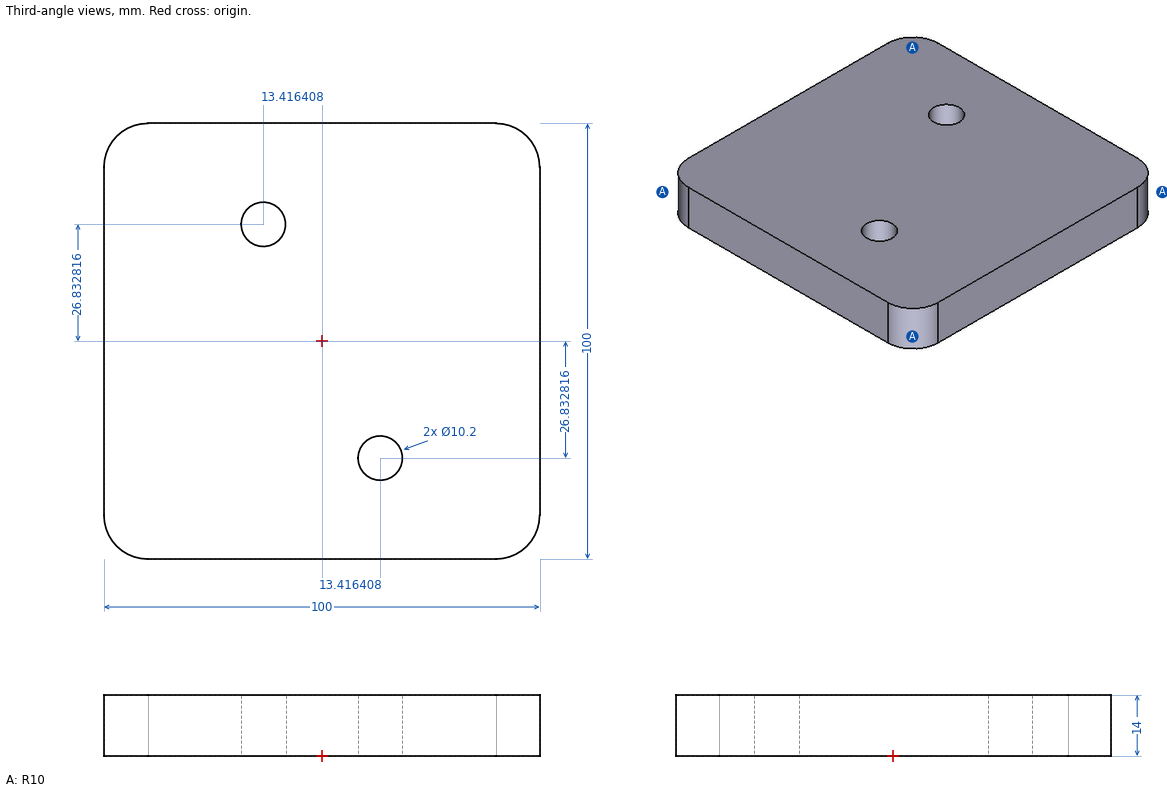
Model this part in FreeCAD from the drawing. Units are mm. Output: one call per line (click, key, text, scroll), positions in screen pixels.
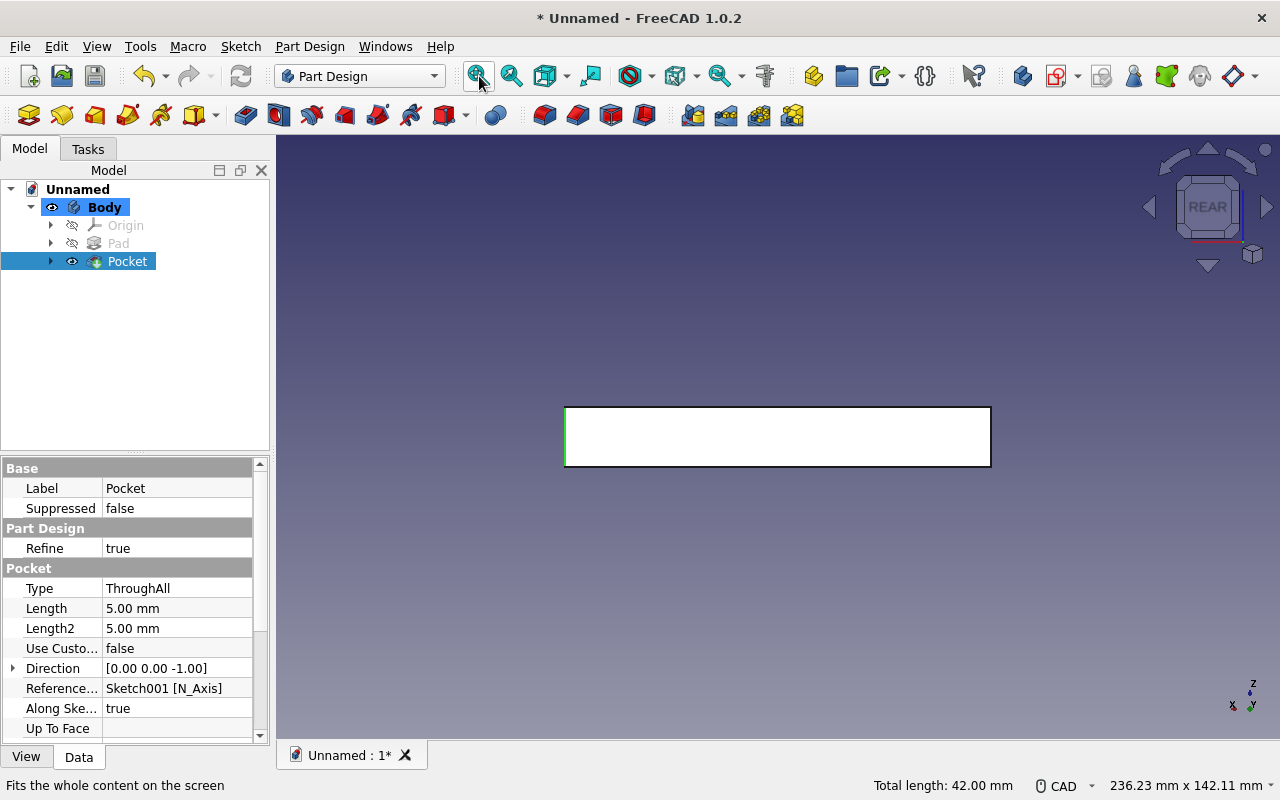
click(991, 436, ctrl)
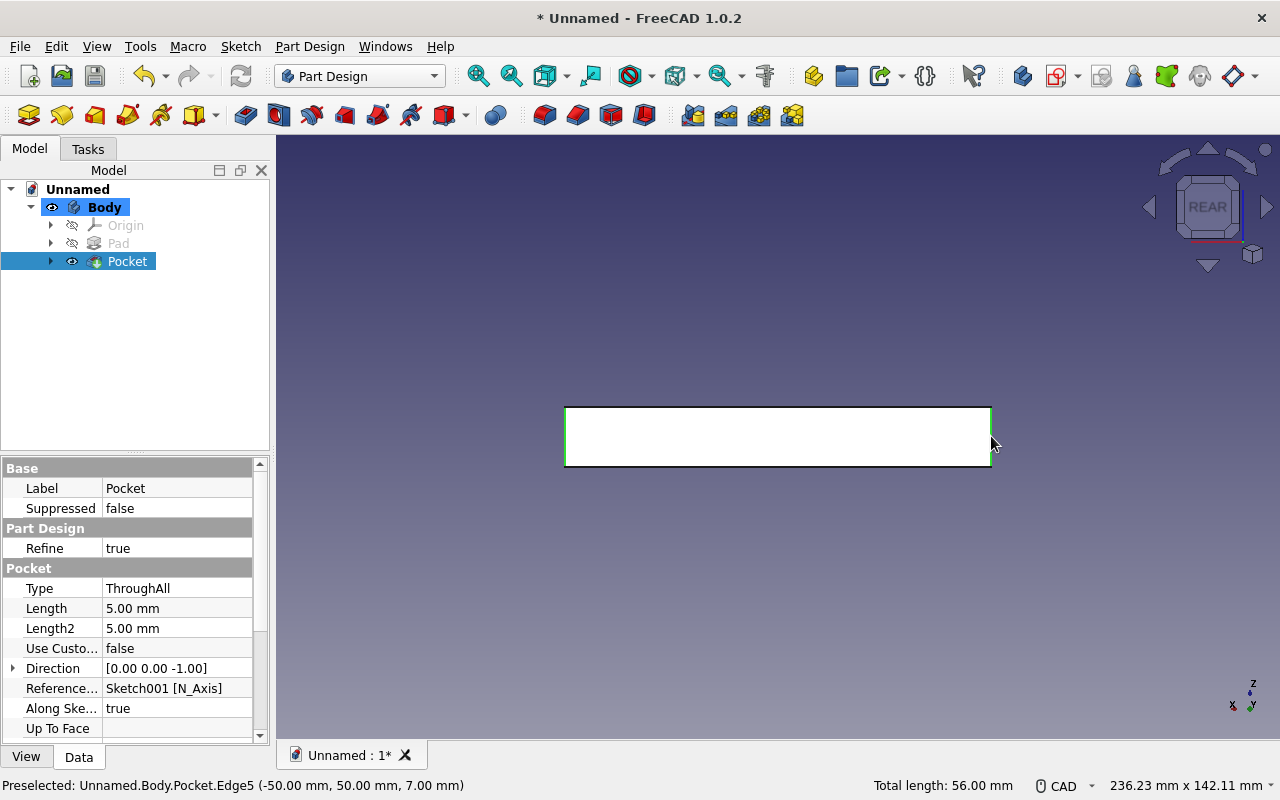
click(545, 116)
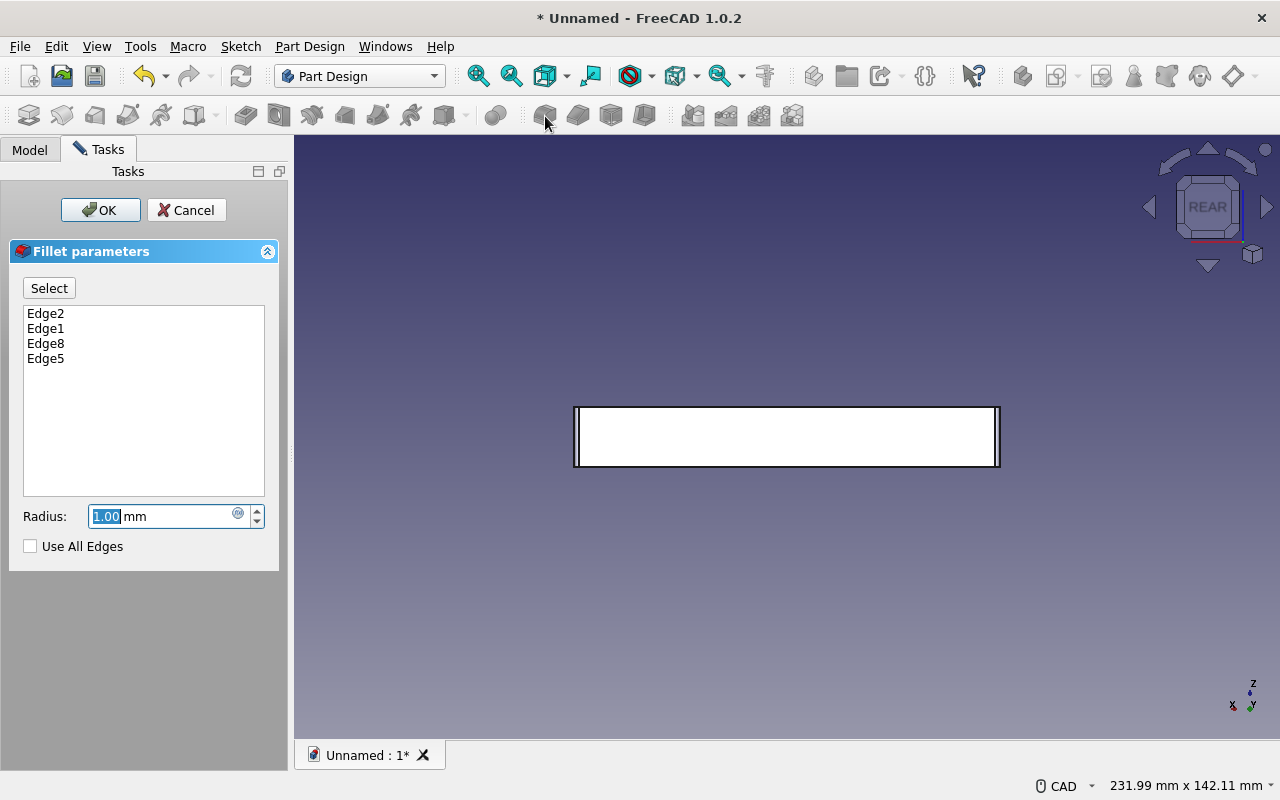
text(10)
key(Tab)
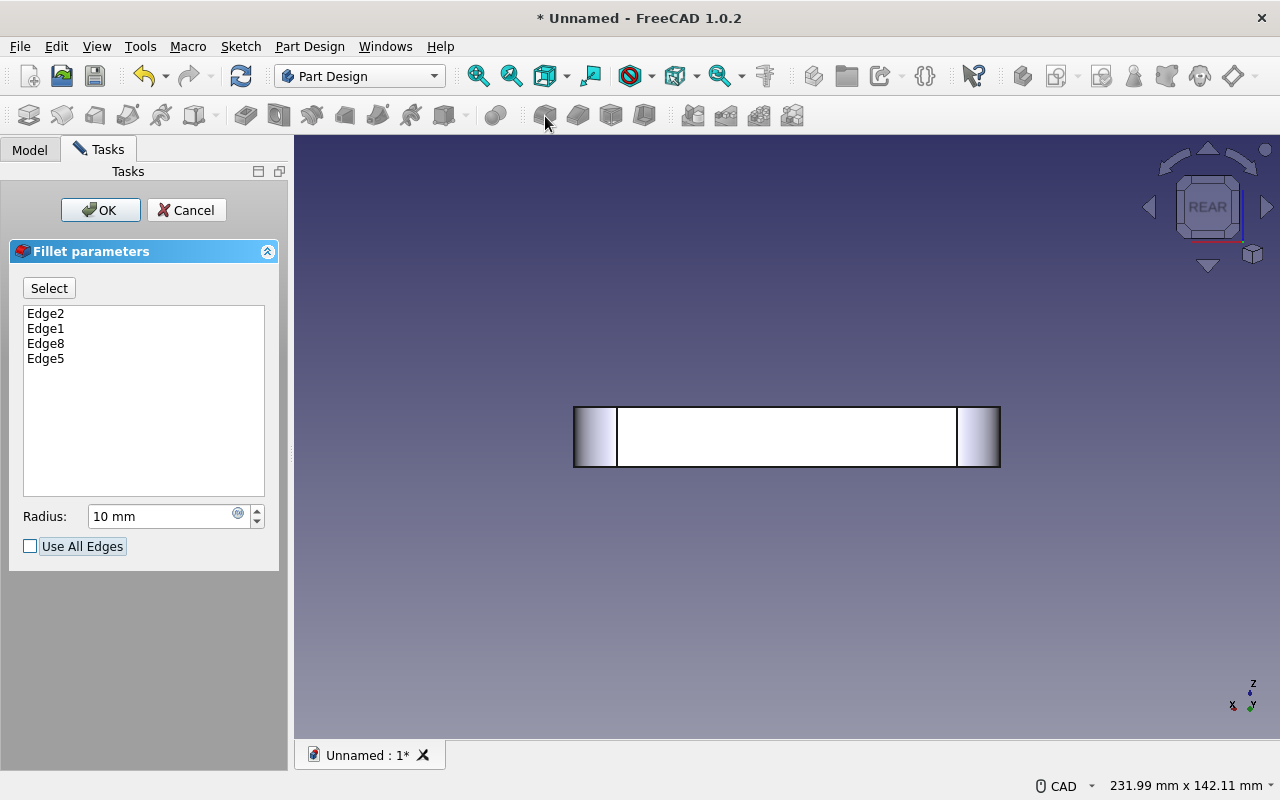
click(101, 210)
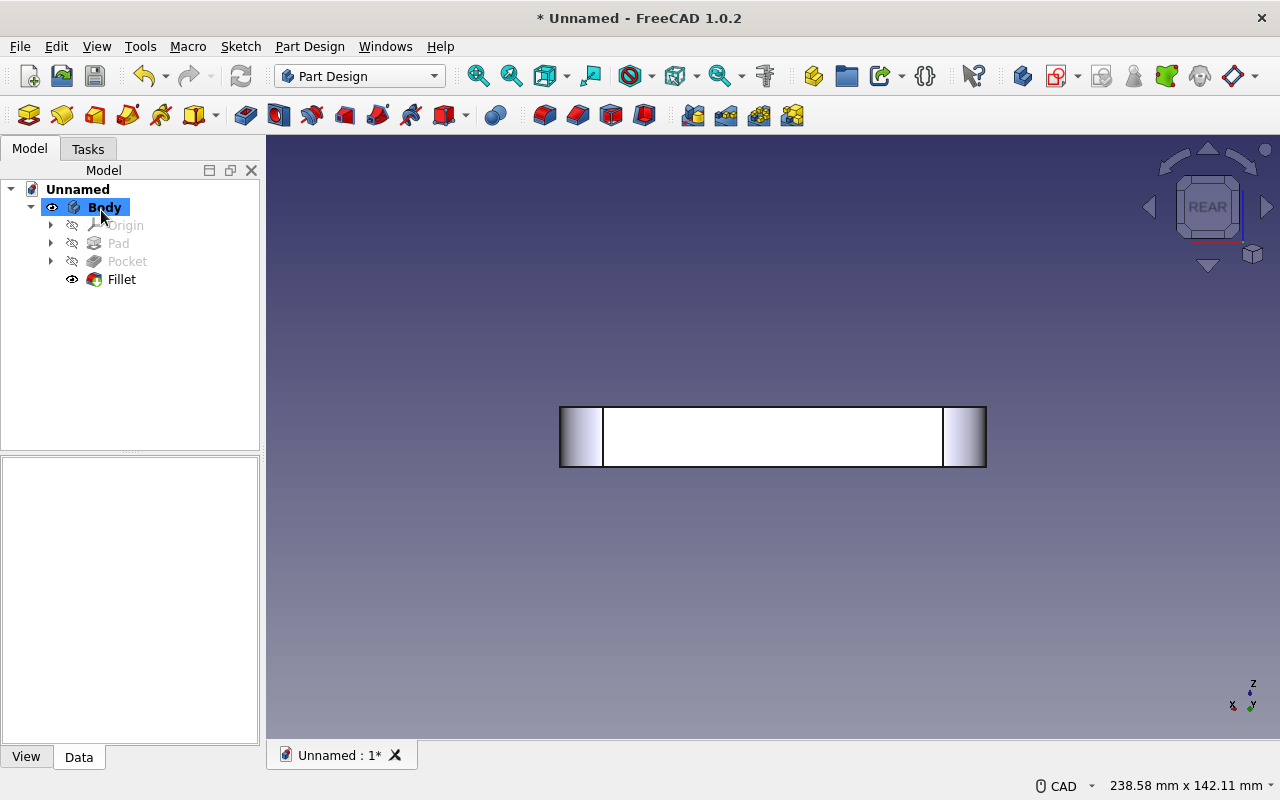
key(0)